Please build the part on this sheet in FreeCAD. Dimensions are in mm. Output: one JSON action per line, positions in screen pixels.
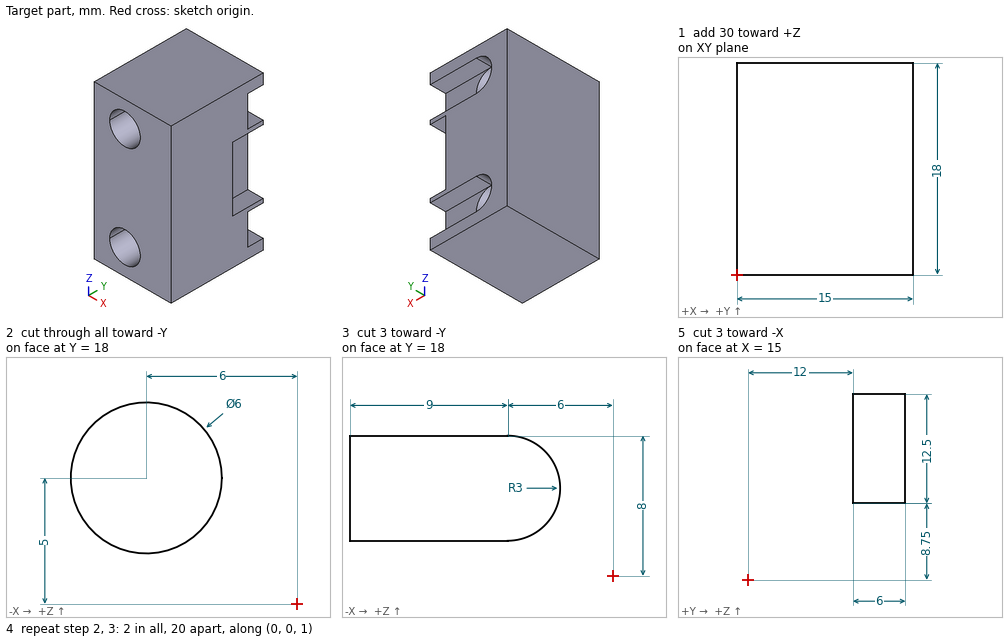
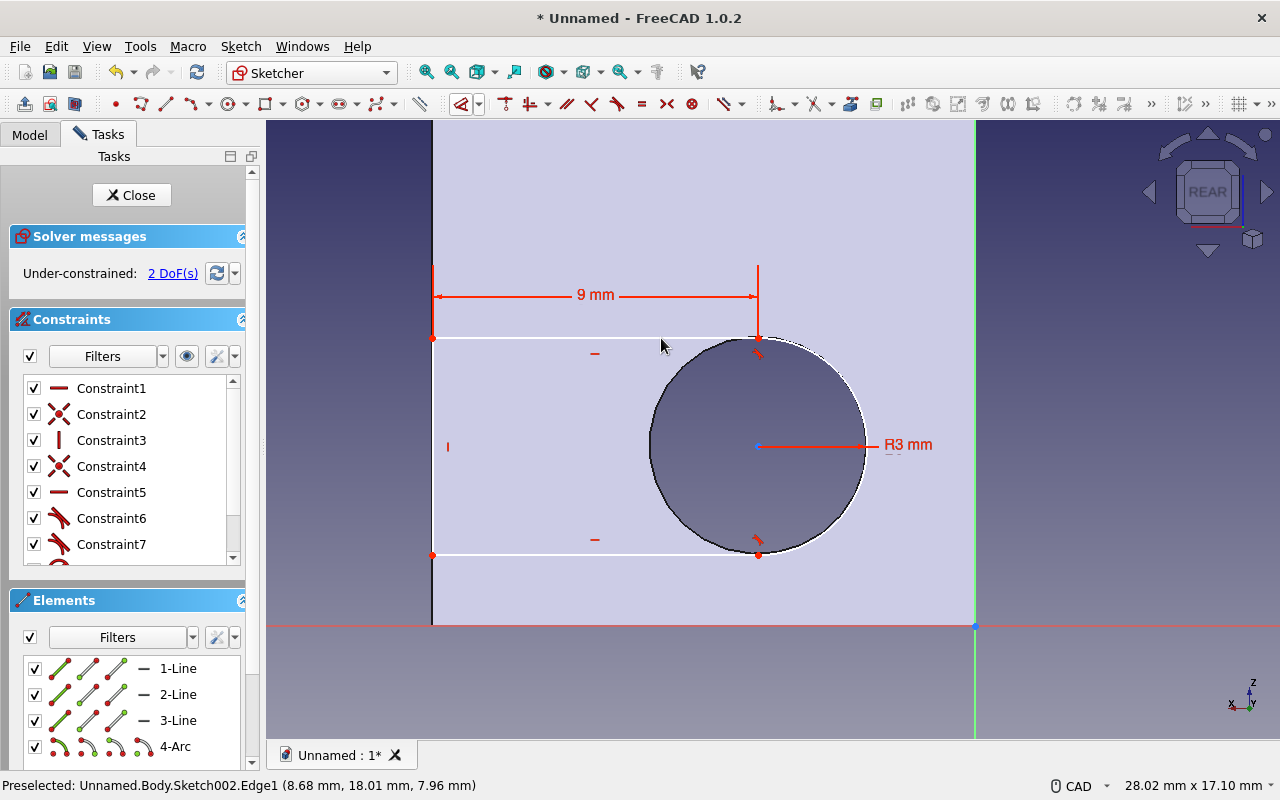
{"action": "left_click", "coordinate": [758, 338]}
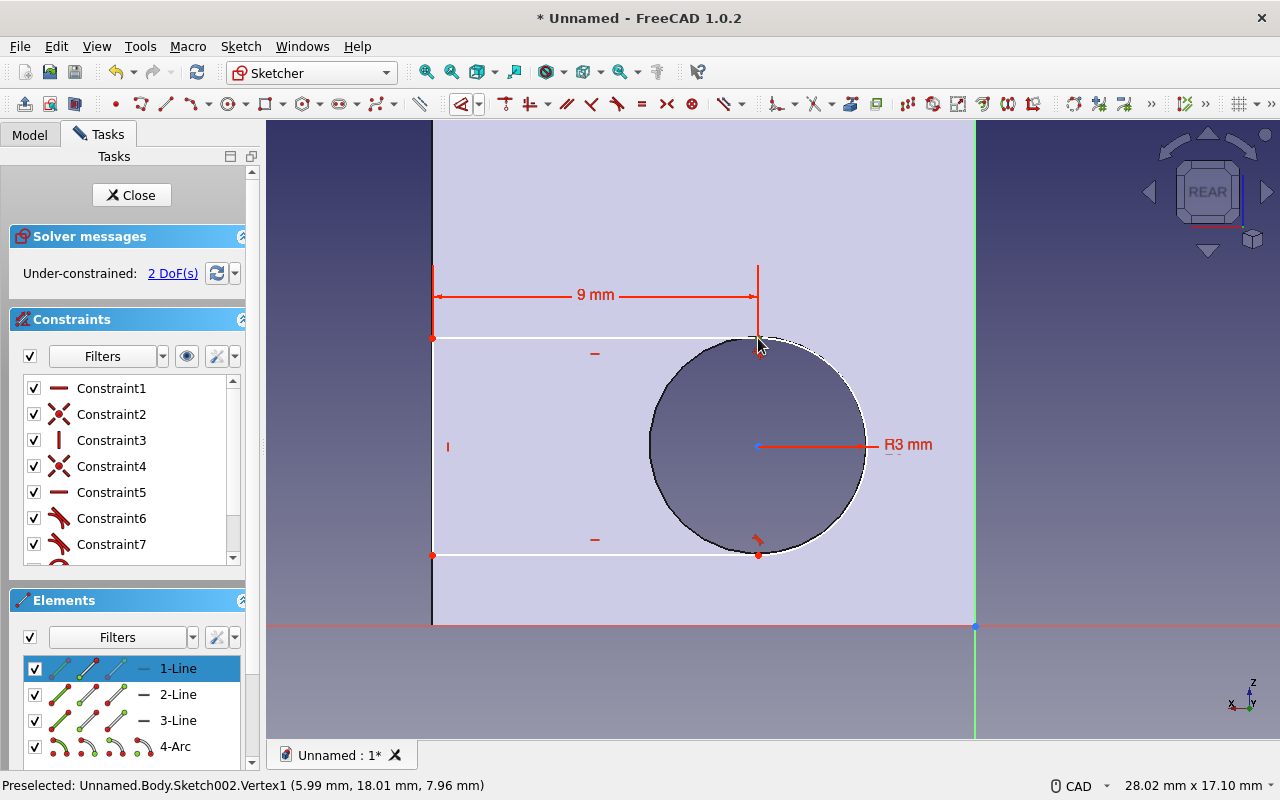
{"action": "key", "text": "l"}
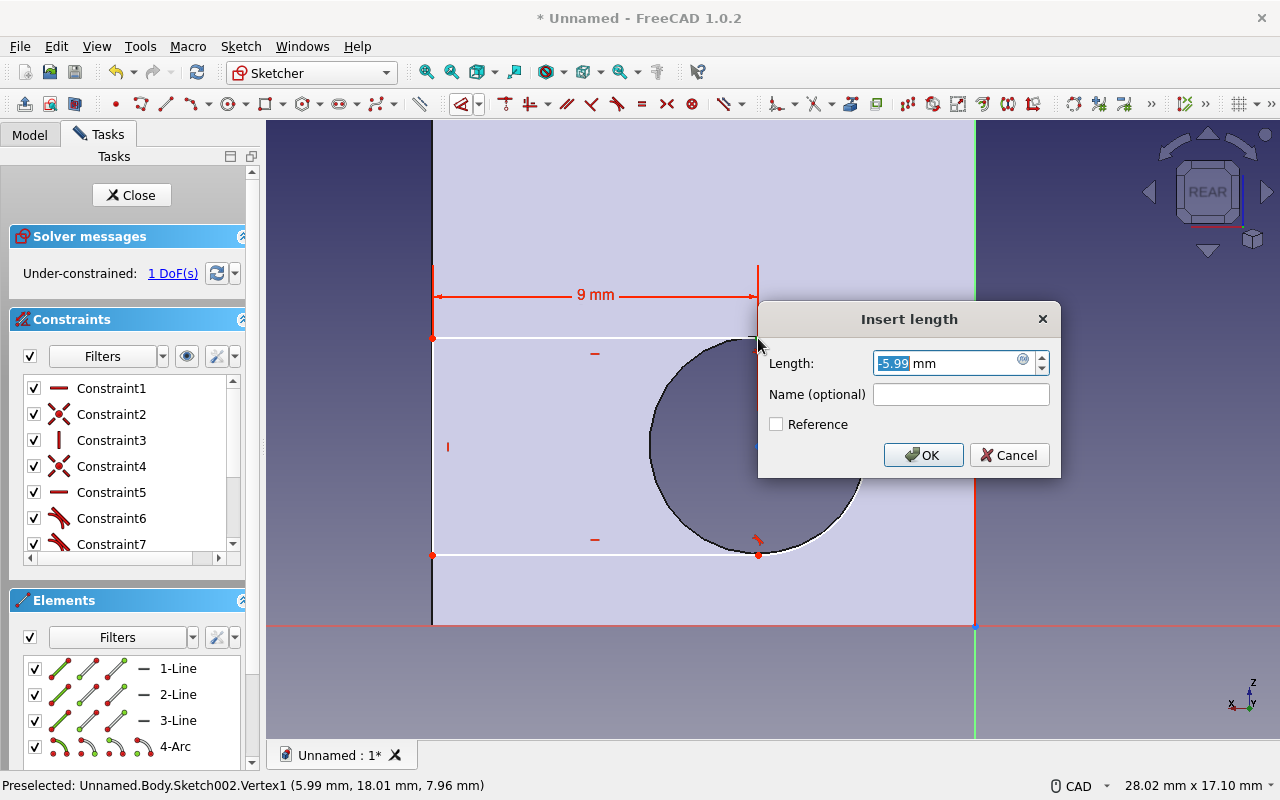
{"action": "type", "text": "-6"}
{"action": "key", "text": "Return"}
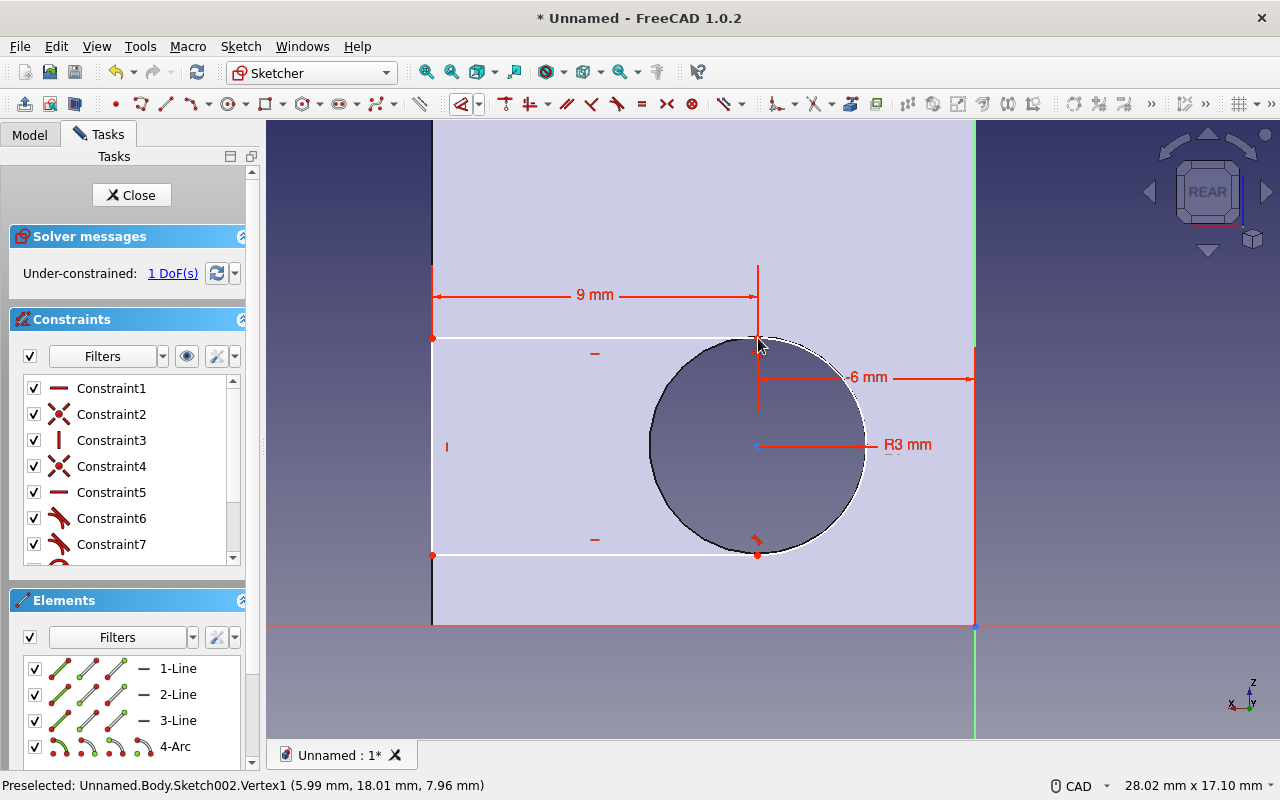
{"action": "left_click", "coordinate": [758, 338]}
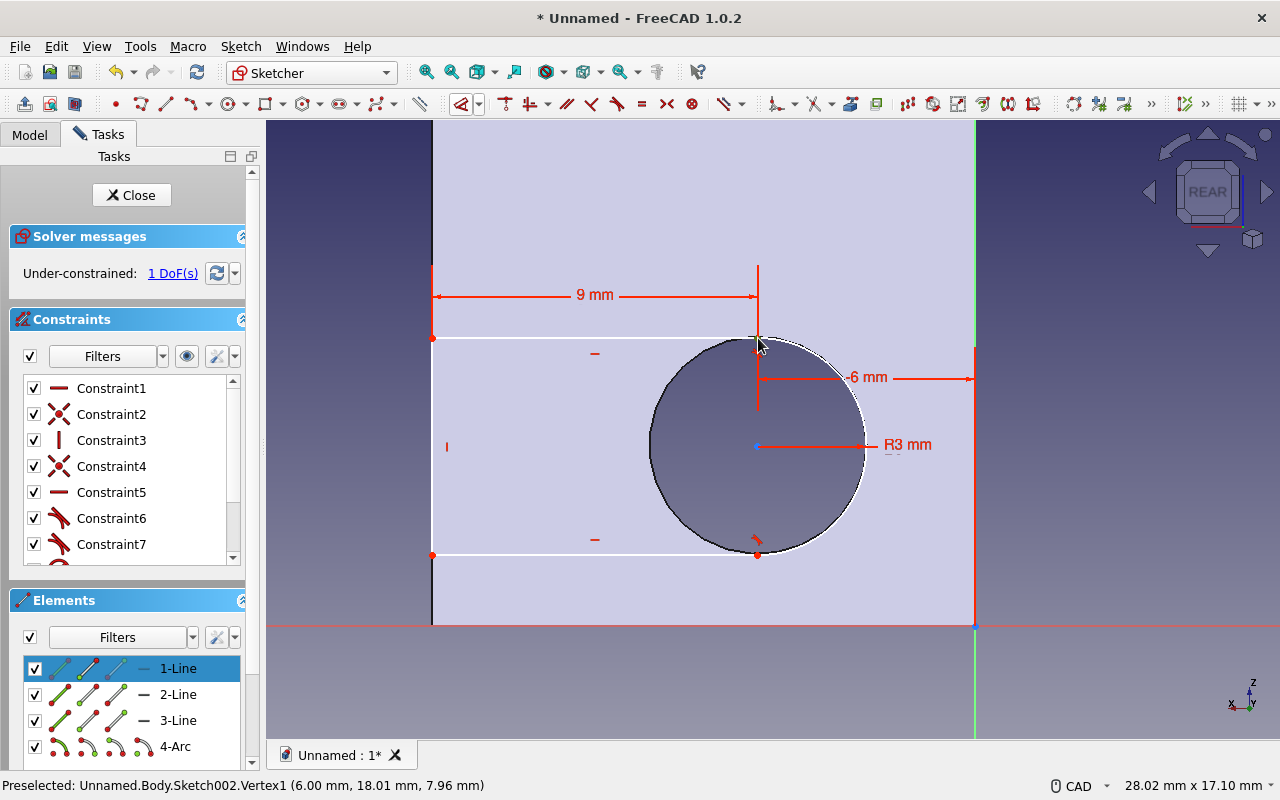
{"action": "left_click", "coordinate": [478, 104]}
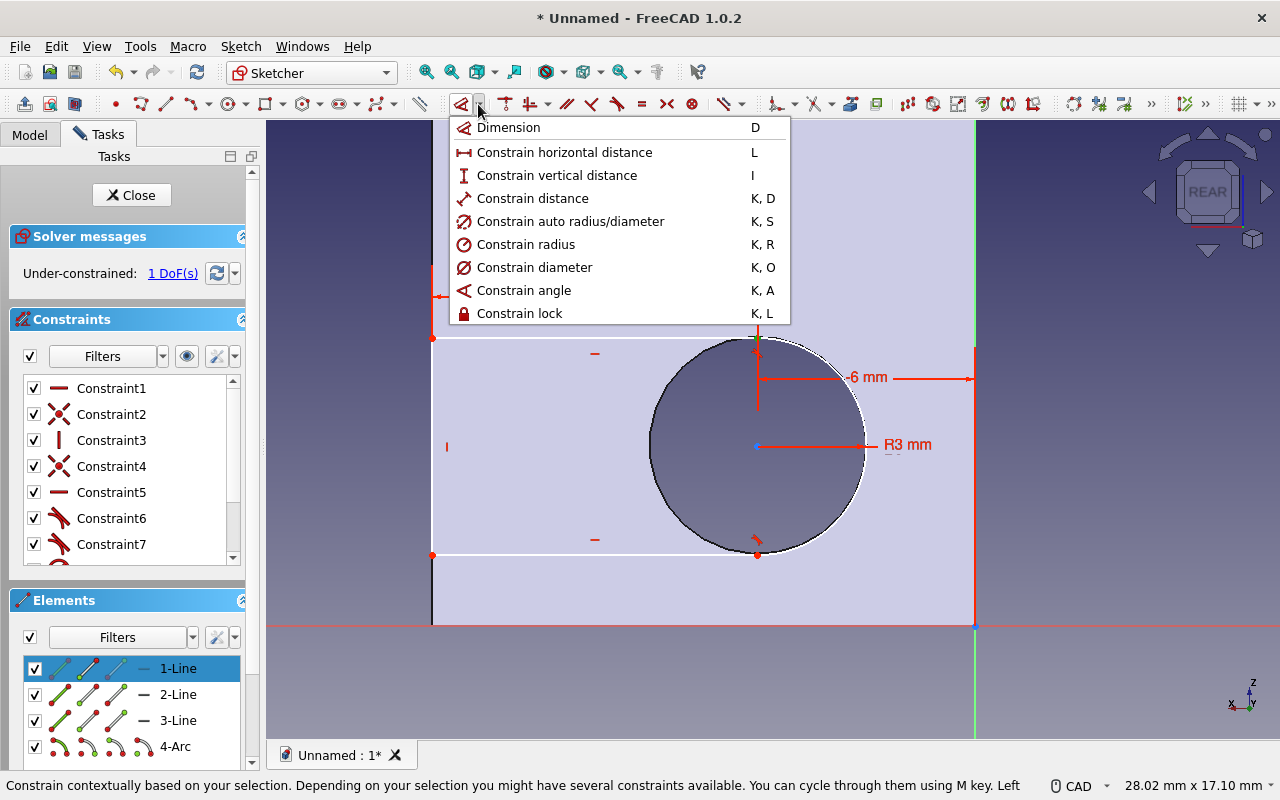
{"action": "left_click", "coordinate": [620, 176]}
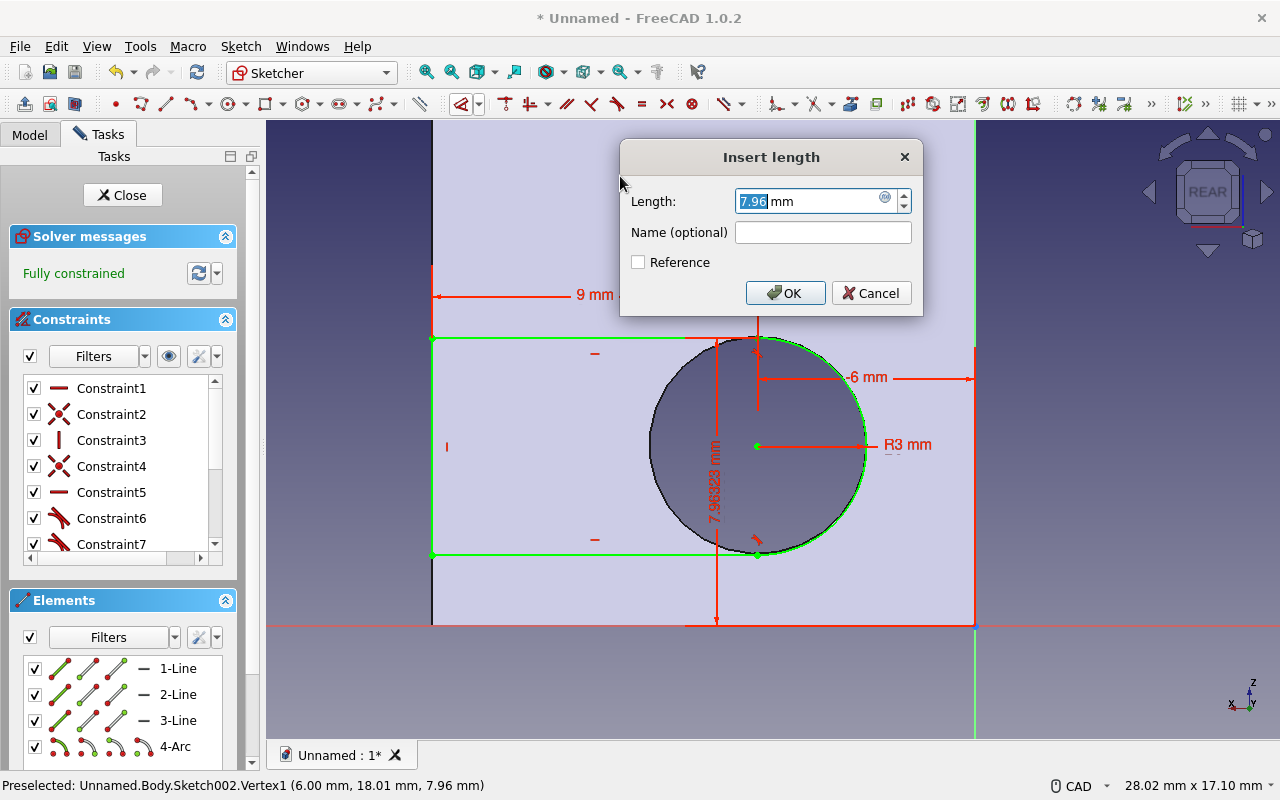
{"action": "type", "text": "8"}
{"action": "key", "text": "Return"}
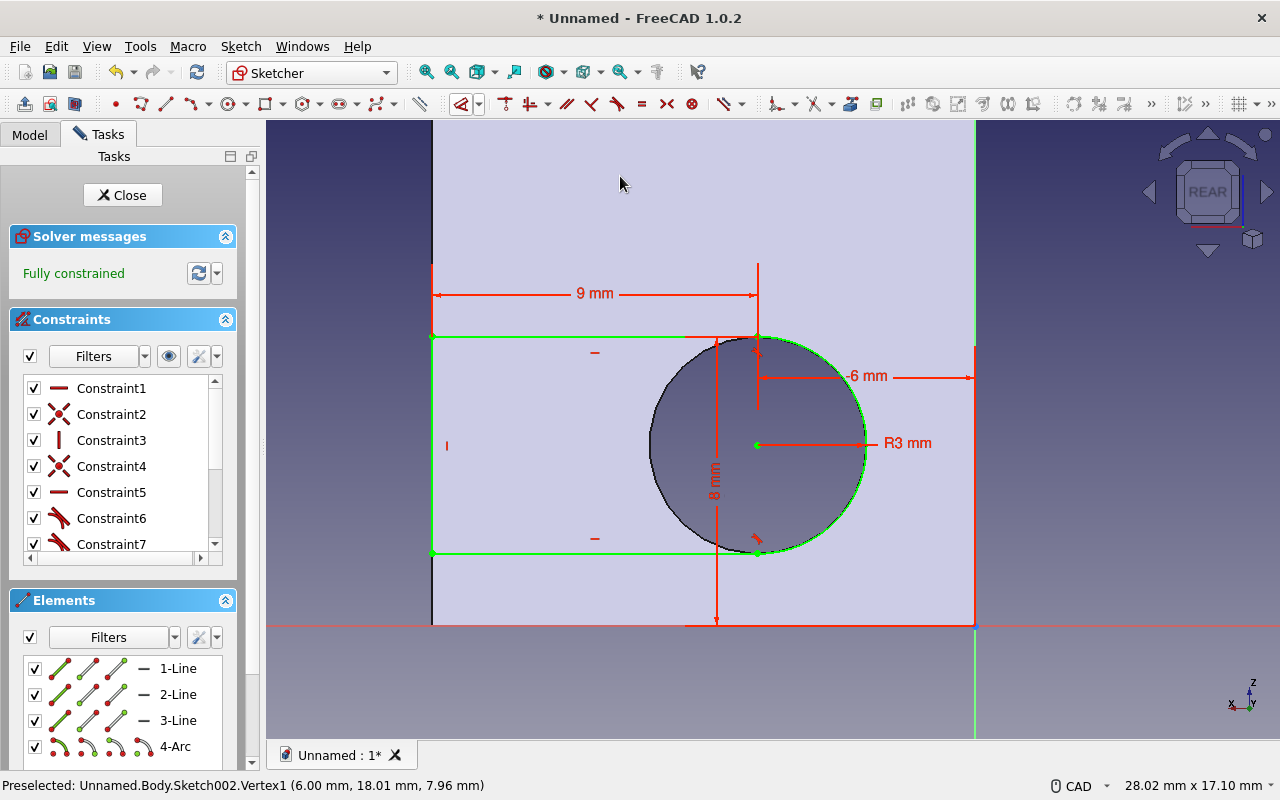
{"action": "left_click", "coordinate": [123, 195]}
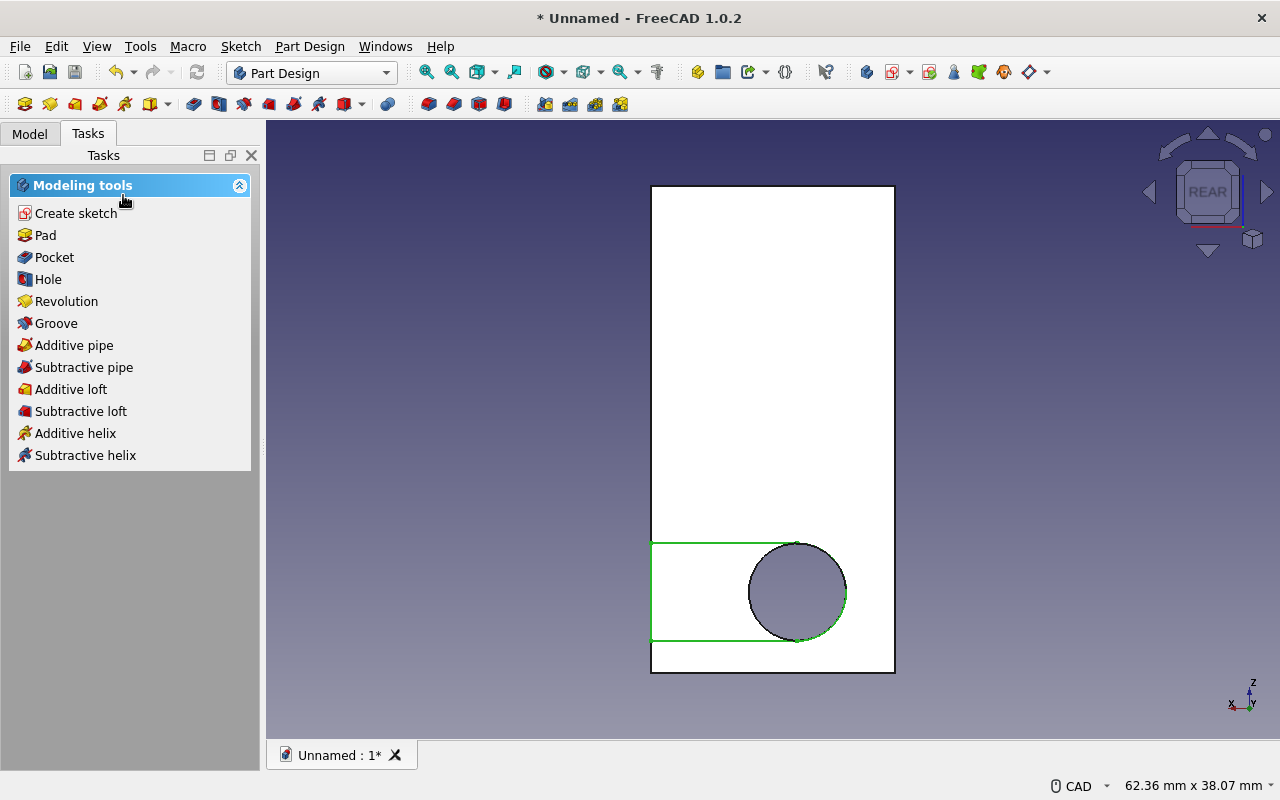
{"action": "left_click", "coordinate": [194, 104]}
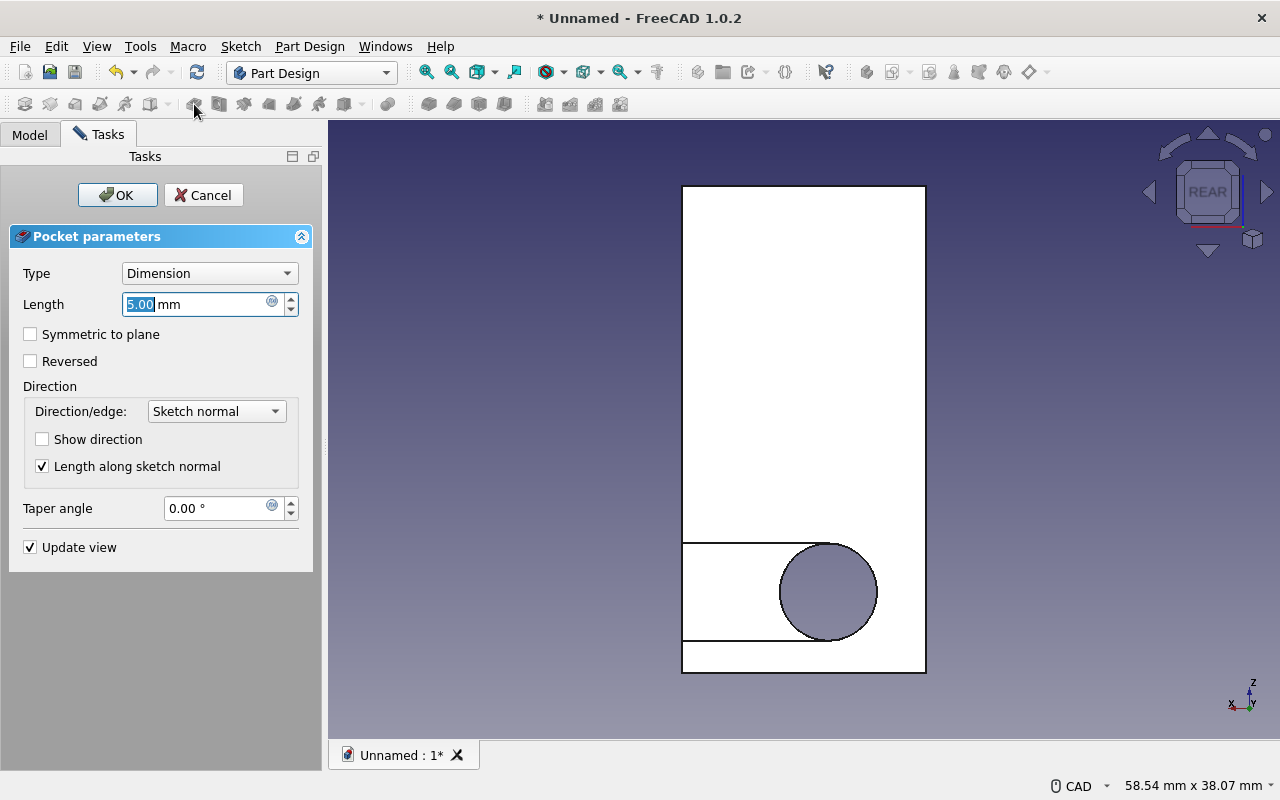
{"action": "type", "text": "3"}
{"action": "key", "text": "Tab"}